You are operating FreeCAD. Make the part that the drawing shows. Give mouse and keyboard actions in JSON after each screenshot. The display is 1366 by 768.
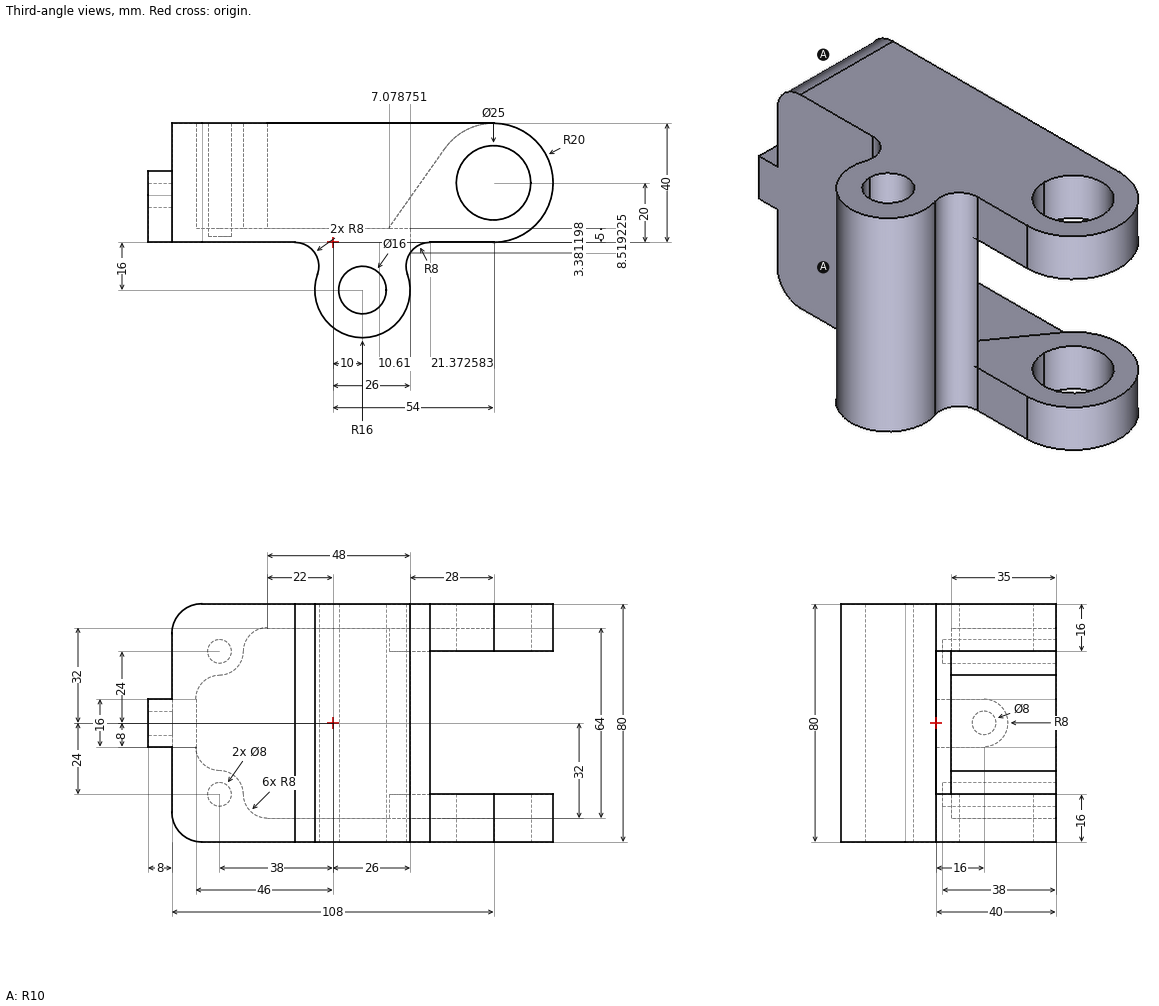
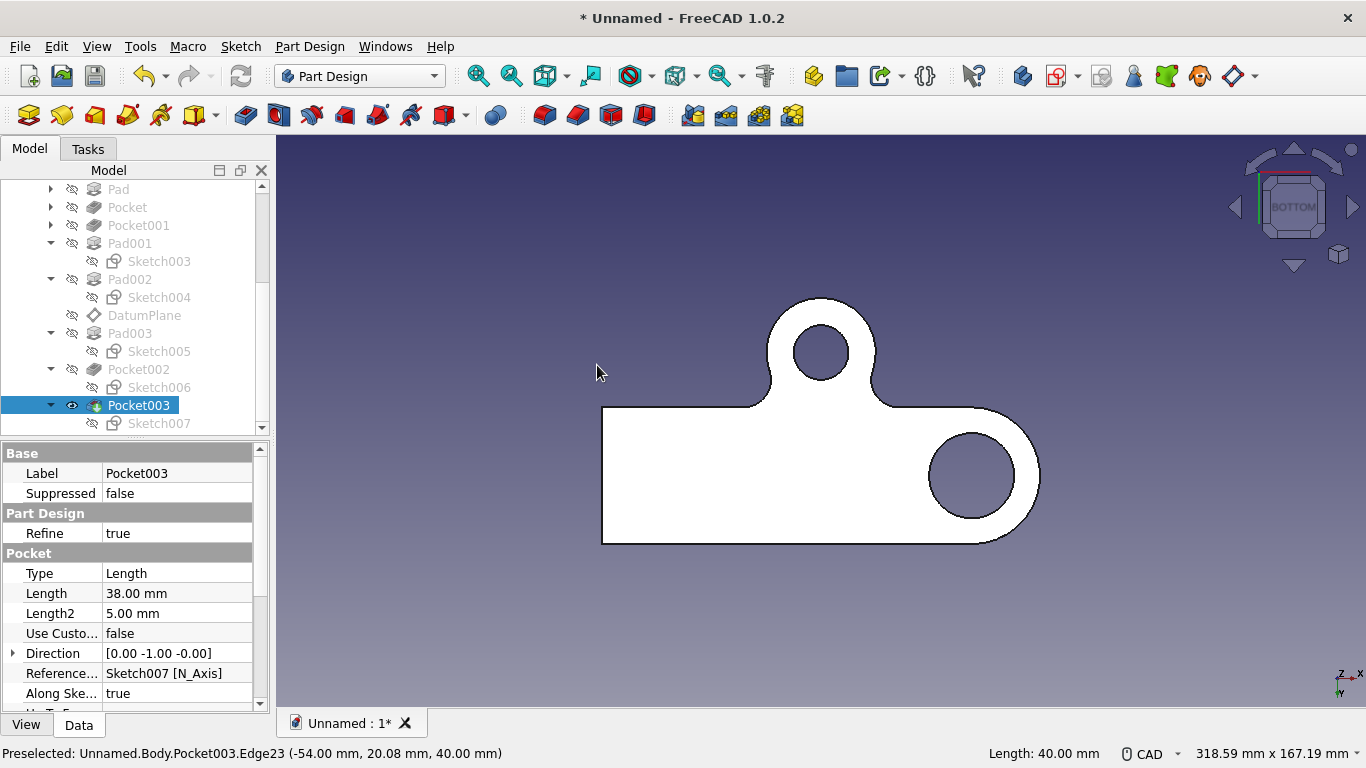
{"action": "left_click", "coordinate": [602, 475], "text": "ctrl"}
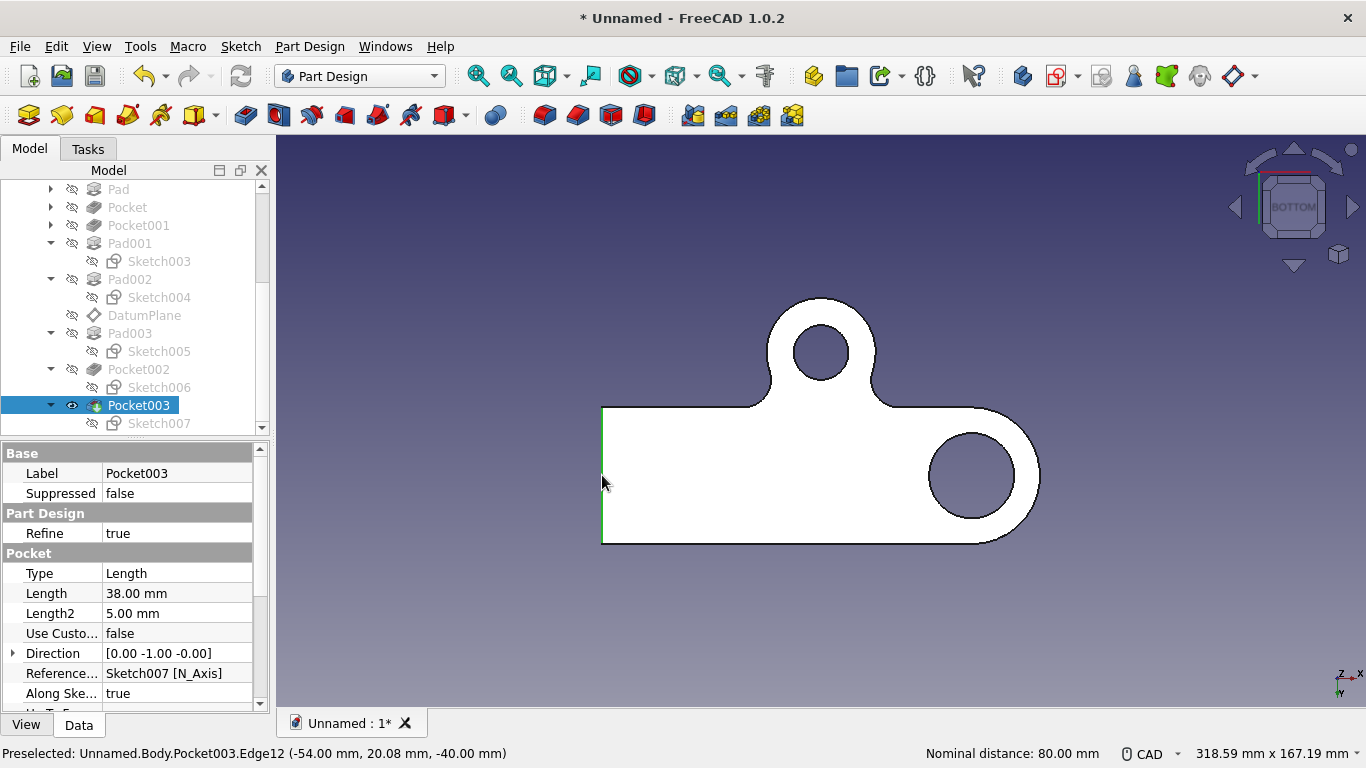
{"action": "left_click", "coordinate": [545, 116]}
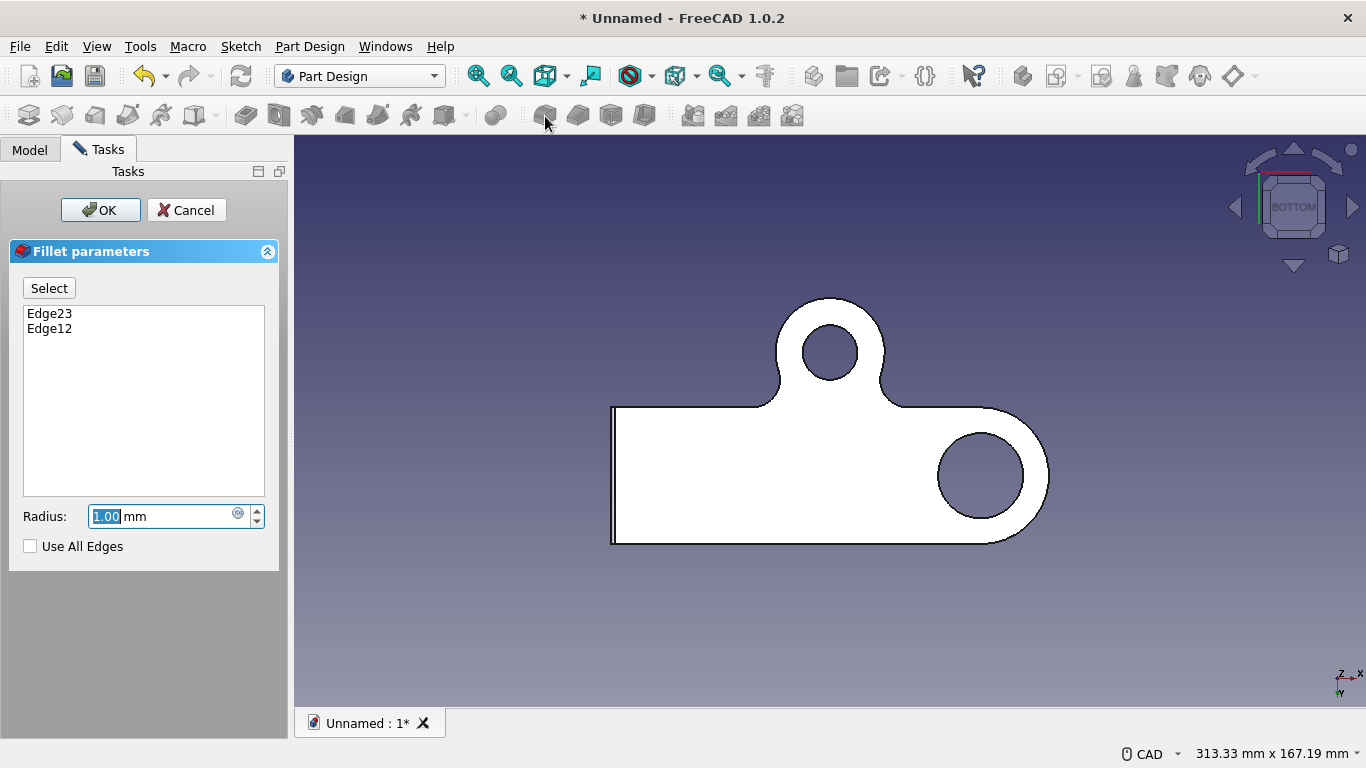
{"action": "type", "text": "10"}
{"action": "key", "text": "Tab"}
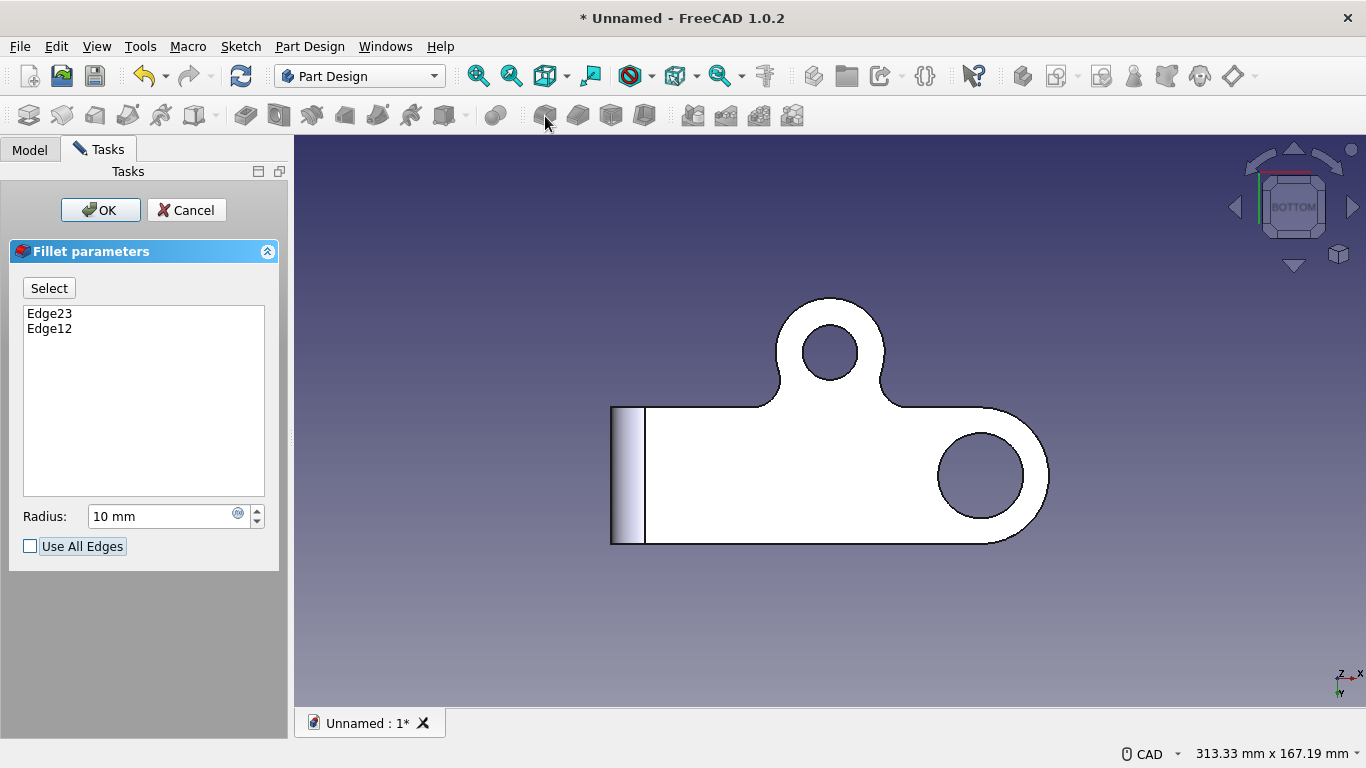
{"action": "left_click", "coordinate": [101, 210]}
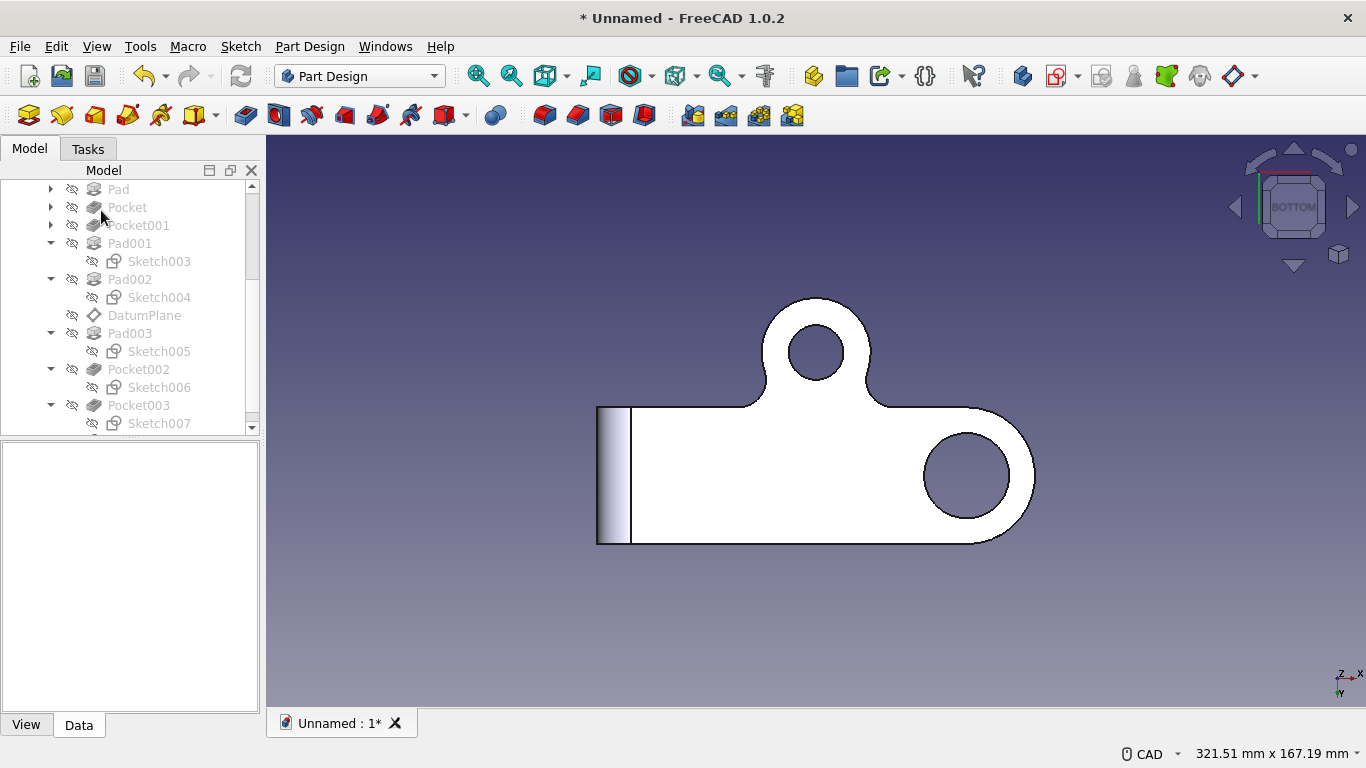
{"action": "key", "text": "v f"}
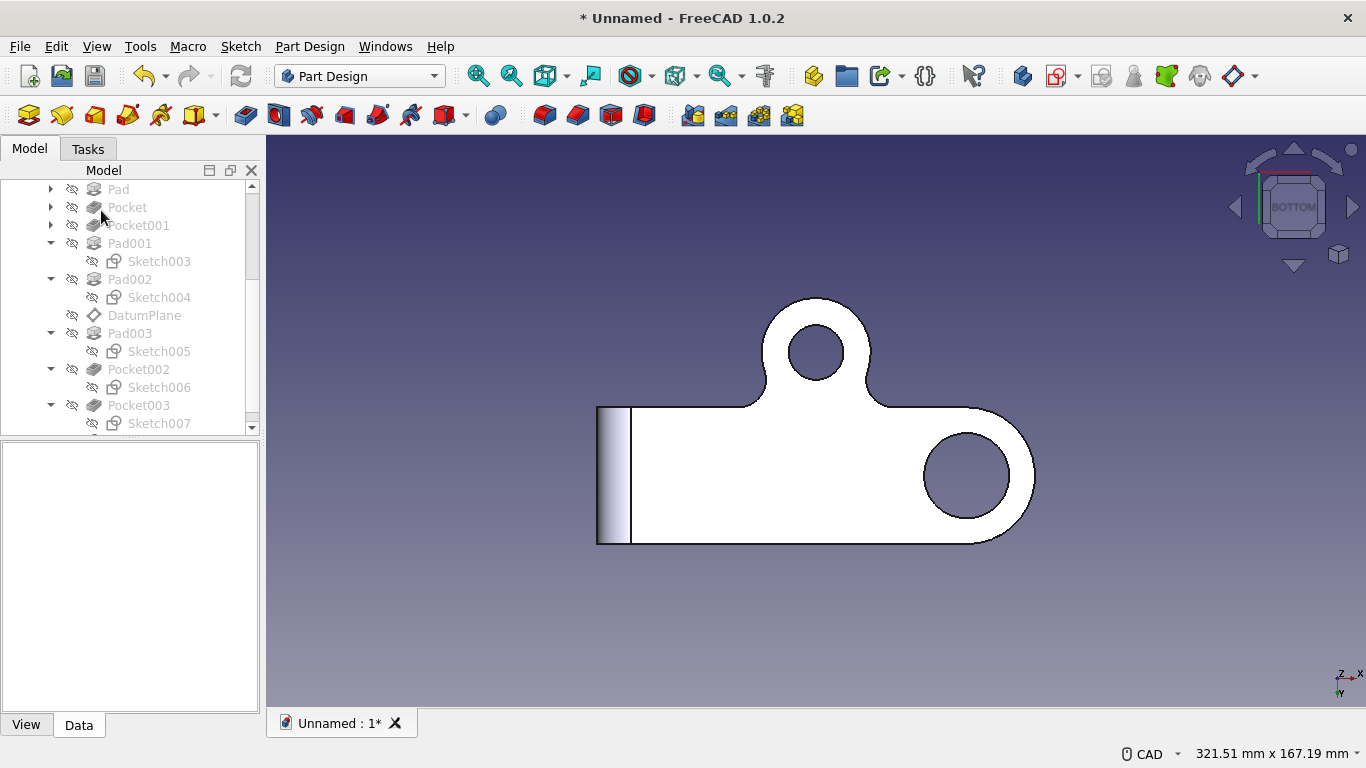
{"action": "key", "text": "6"}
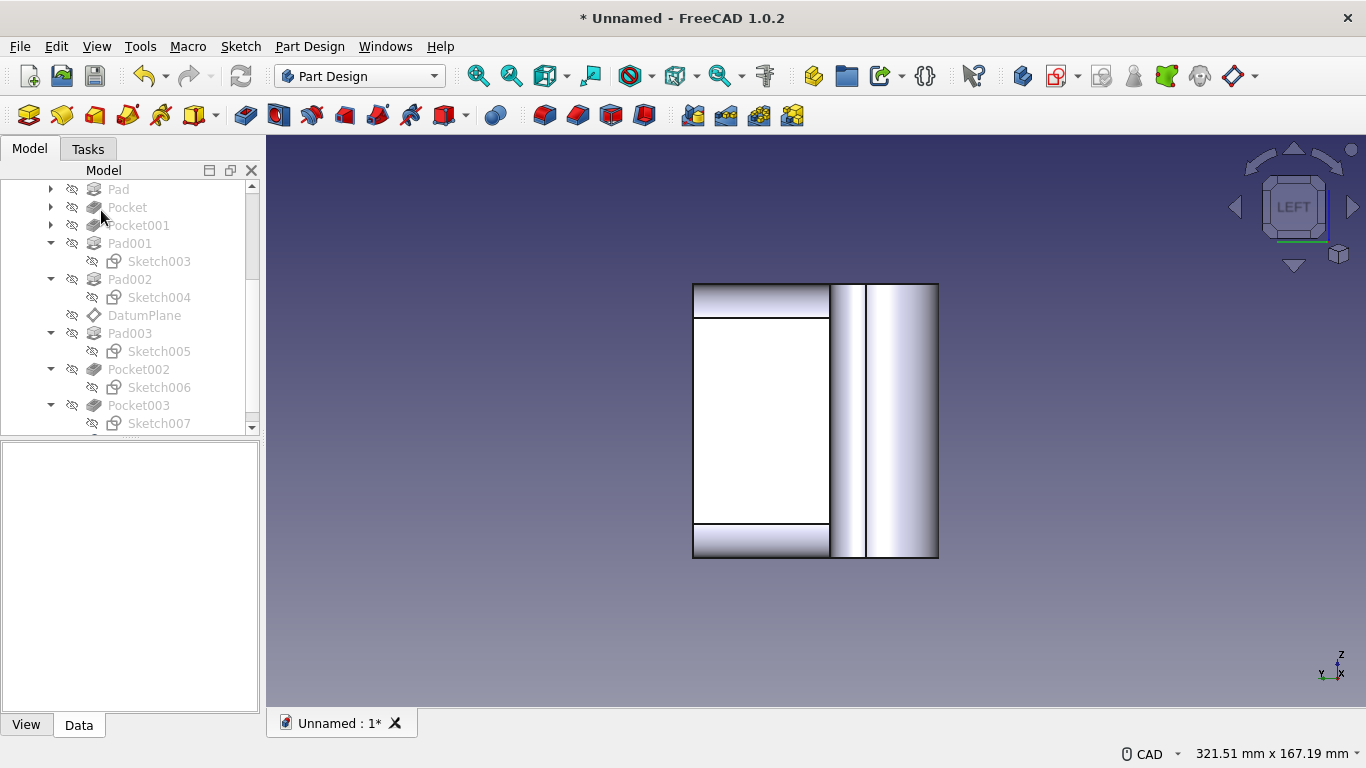
{"action": "left_click", "coordinate": [761, 391]}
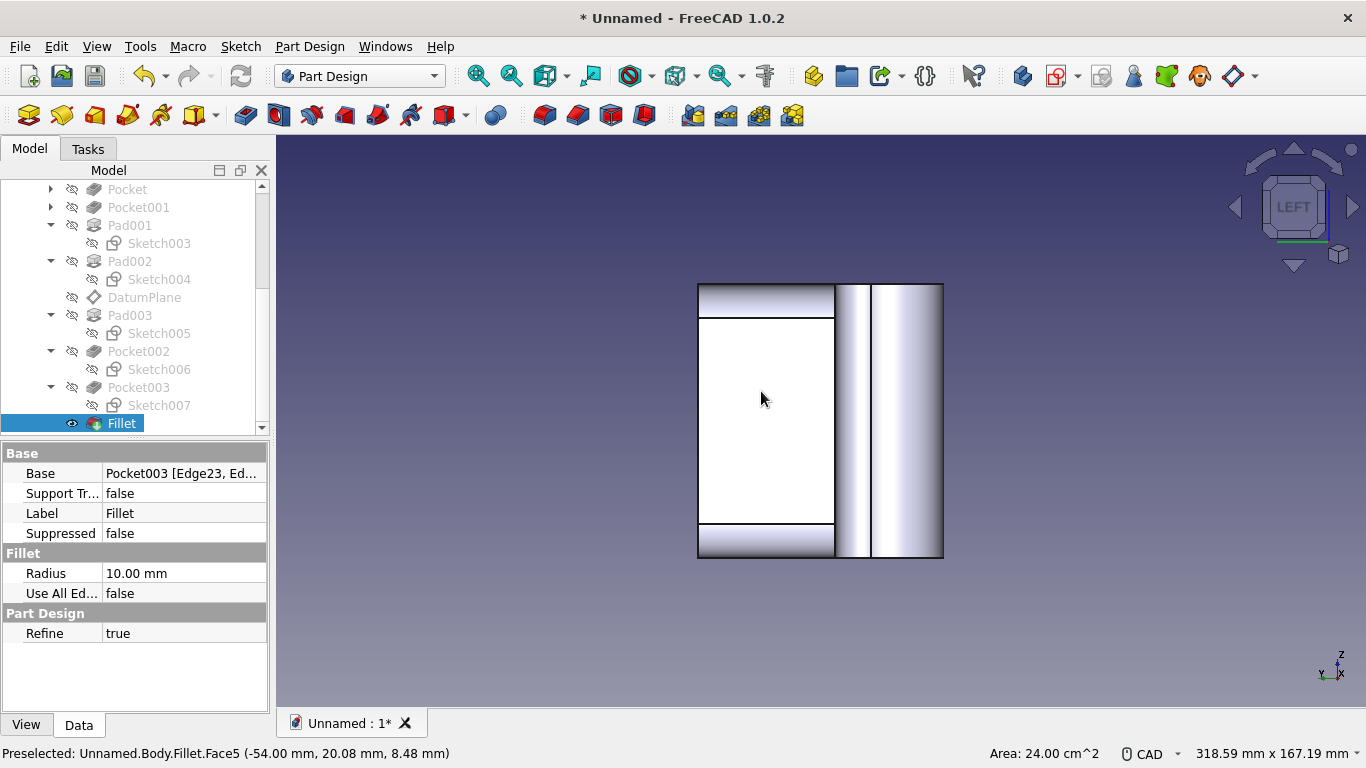
{"action": "left_click", "coordinate": [1056, 76]}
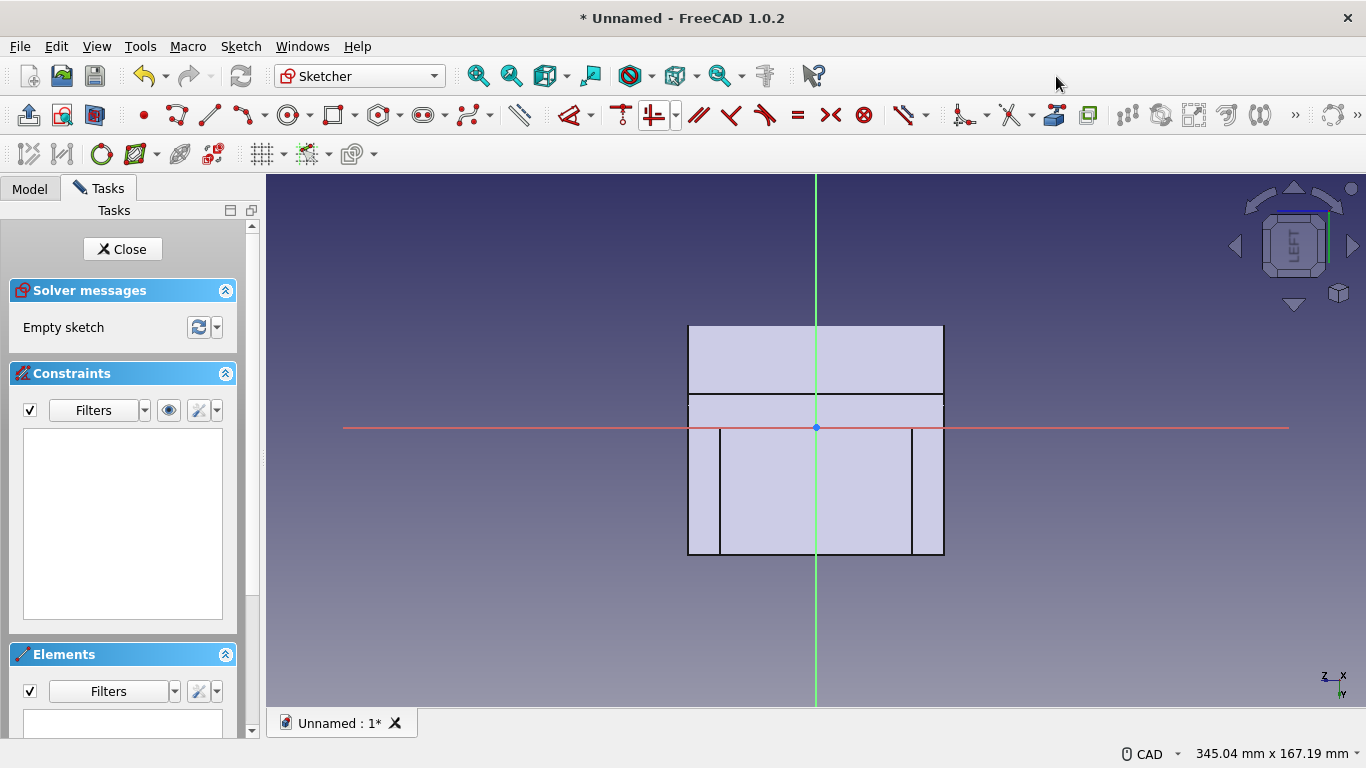
{"action": "scroll", "coordinate": [838, 474], "scroll_direction": "up", "scroll_amount": 7}